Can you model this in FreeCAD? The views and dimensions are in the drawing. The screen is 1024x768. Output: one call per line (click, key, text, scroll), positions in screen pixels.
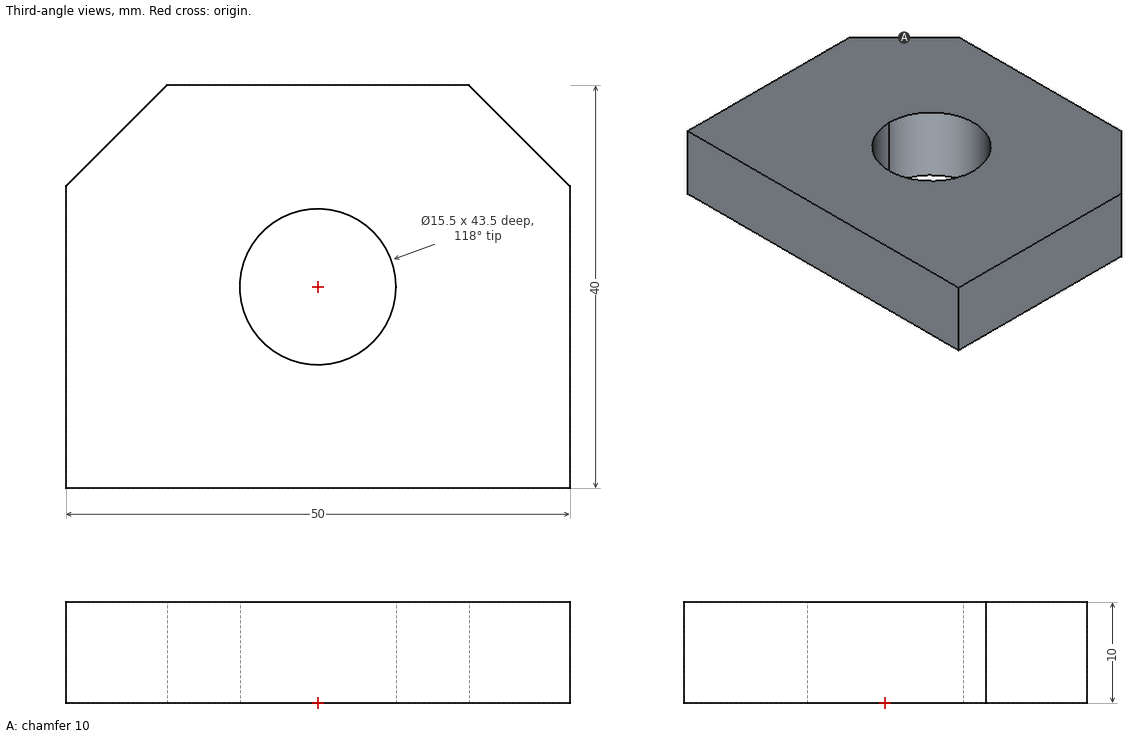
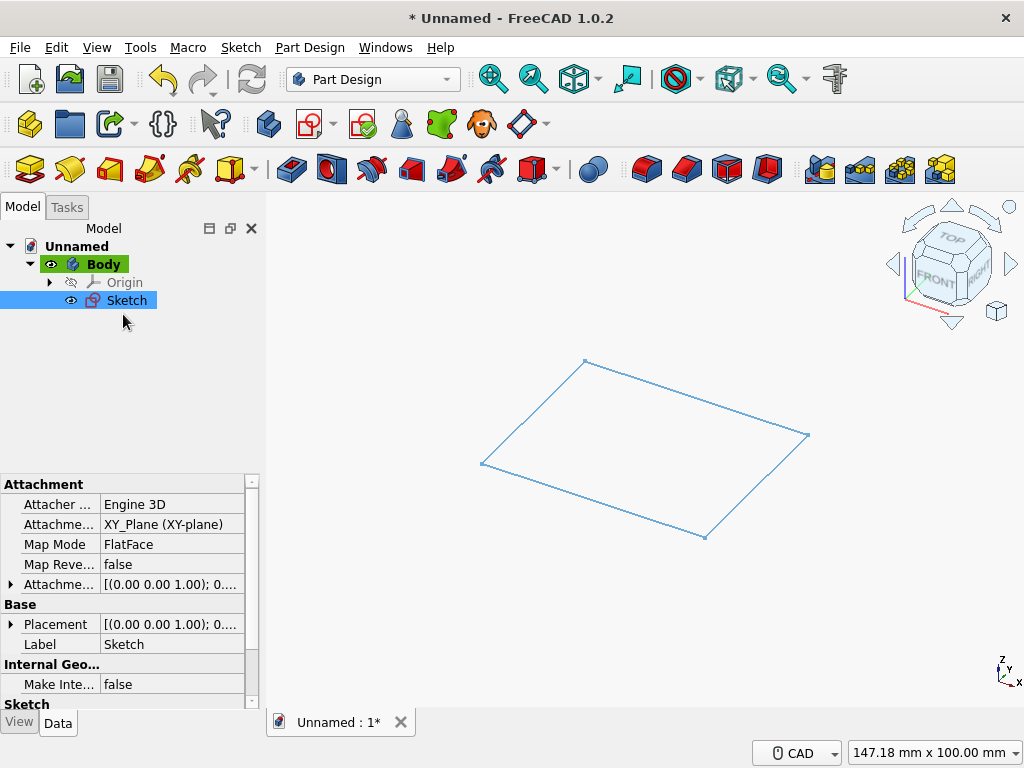
click(30, 170)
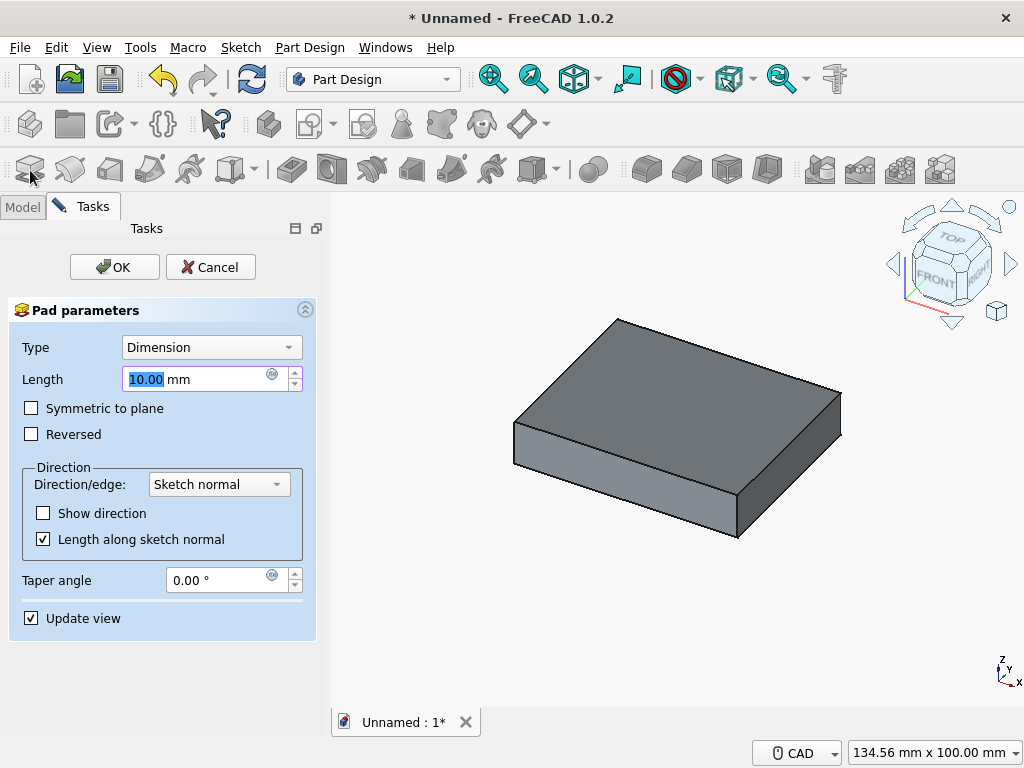
text(10)
key(Tab)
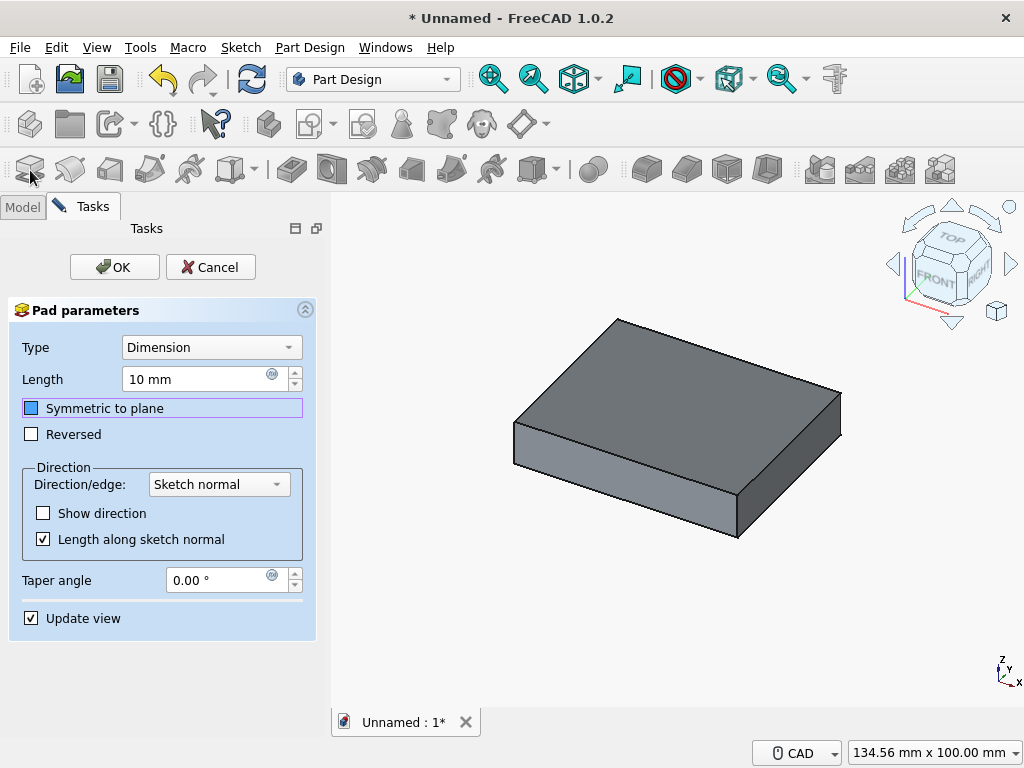
click(115, 267)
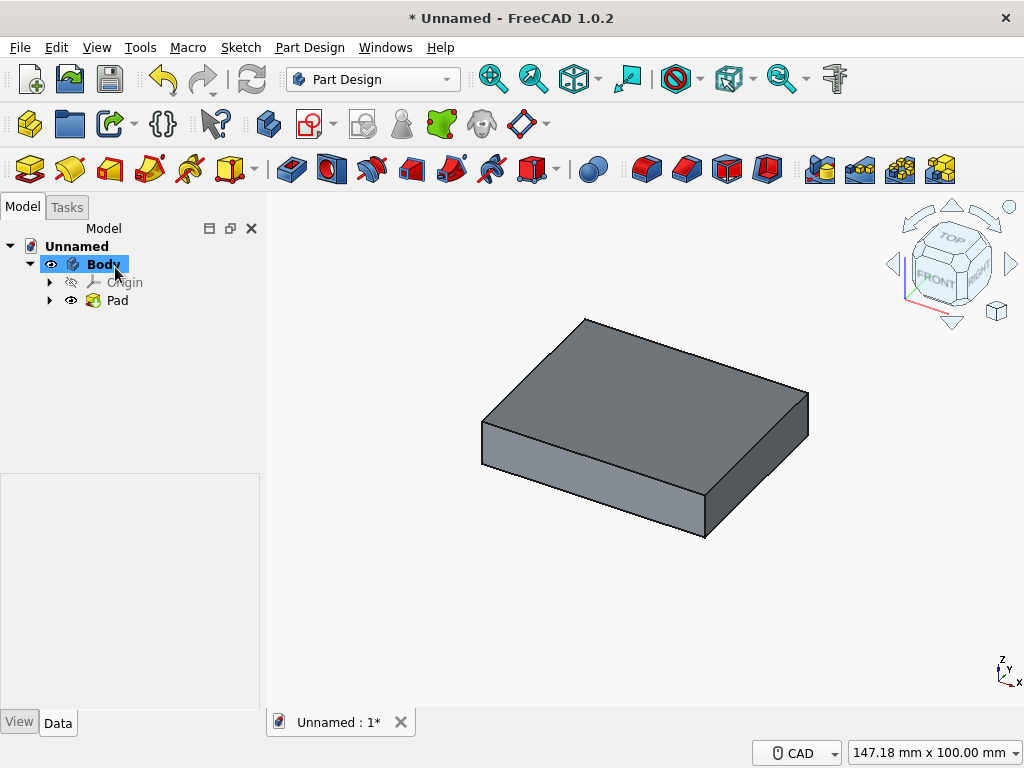
key(v)
key(f)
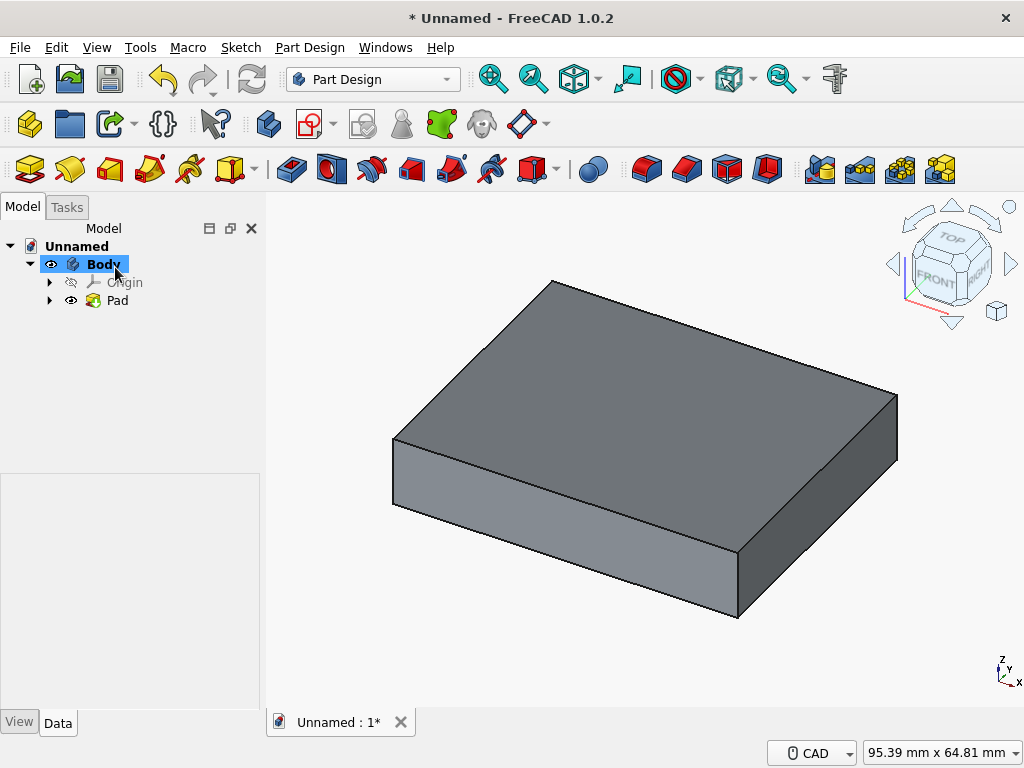
key(0)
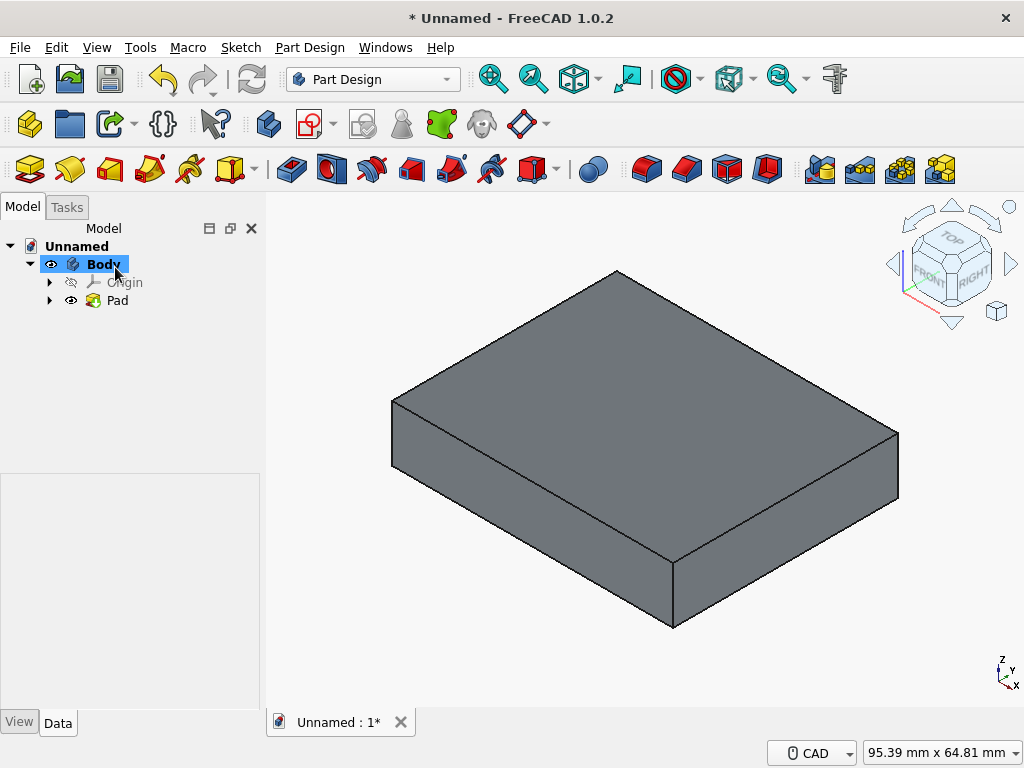
key(2)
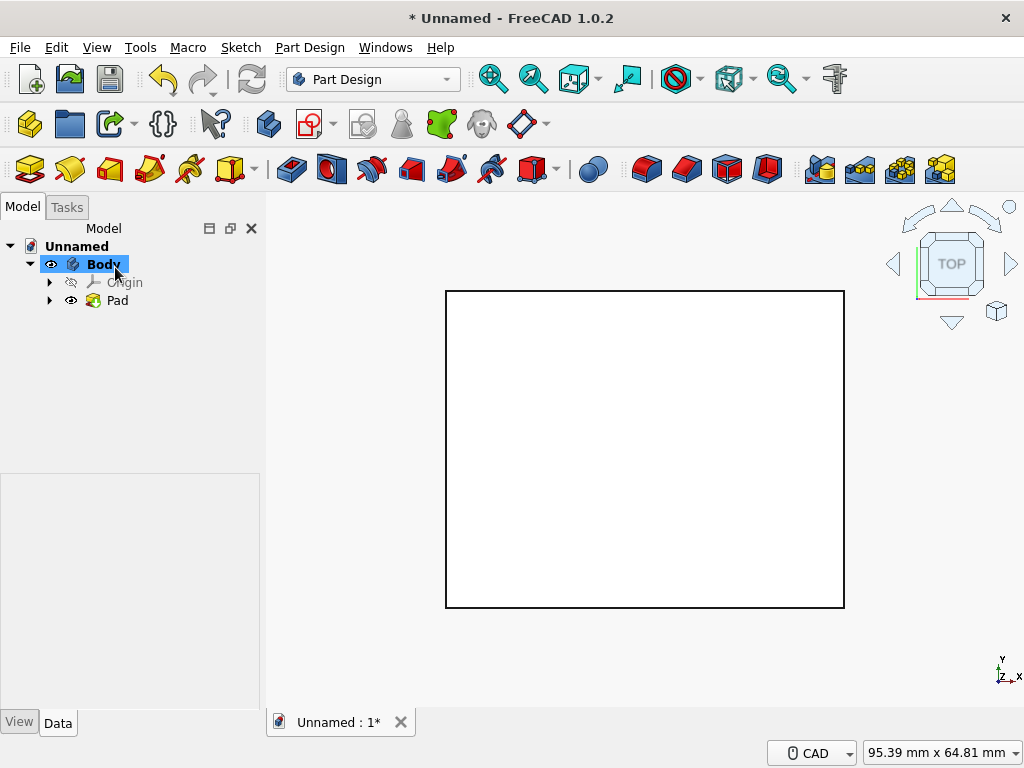
key(1)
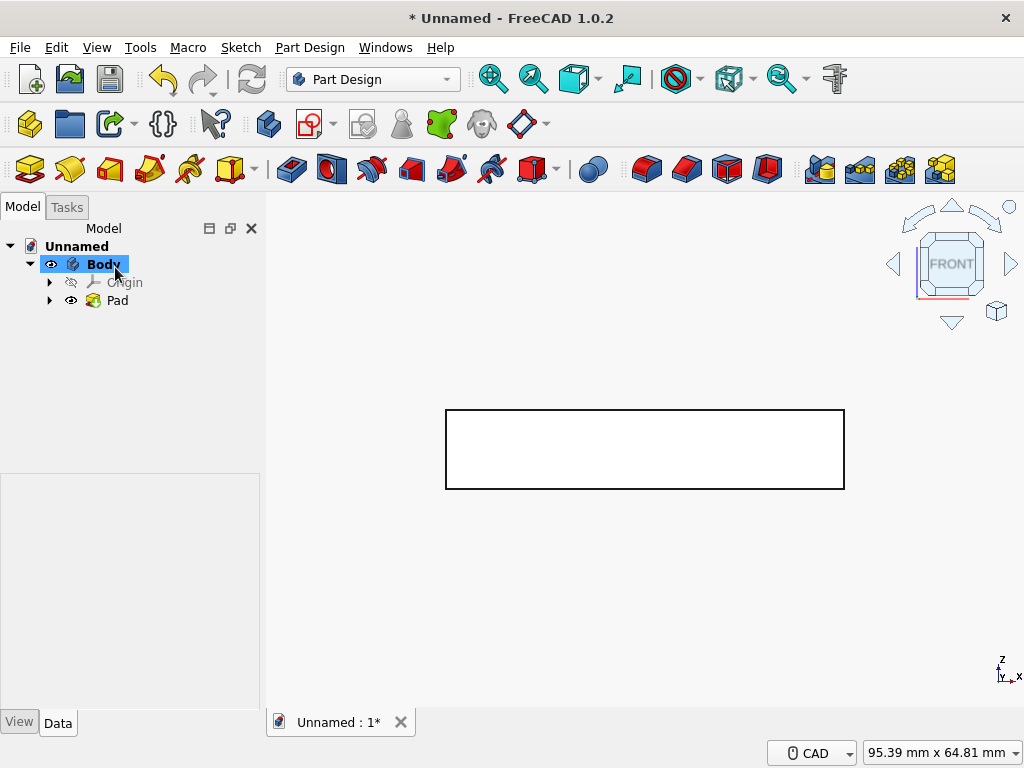
key(3)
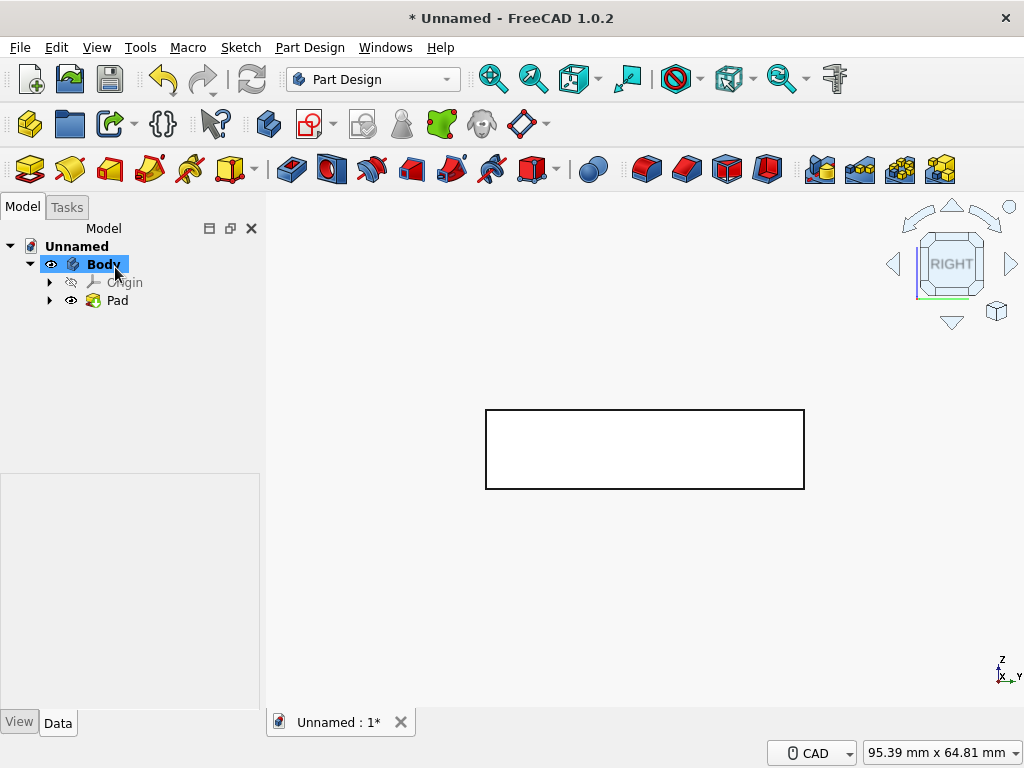
key(v)
key(f)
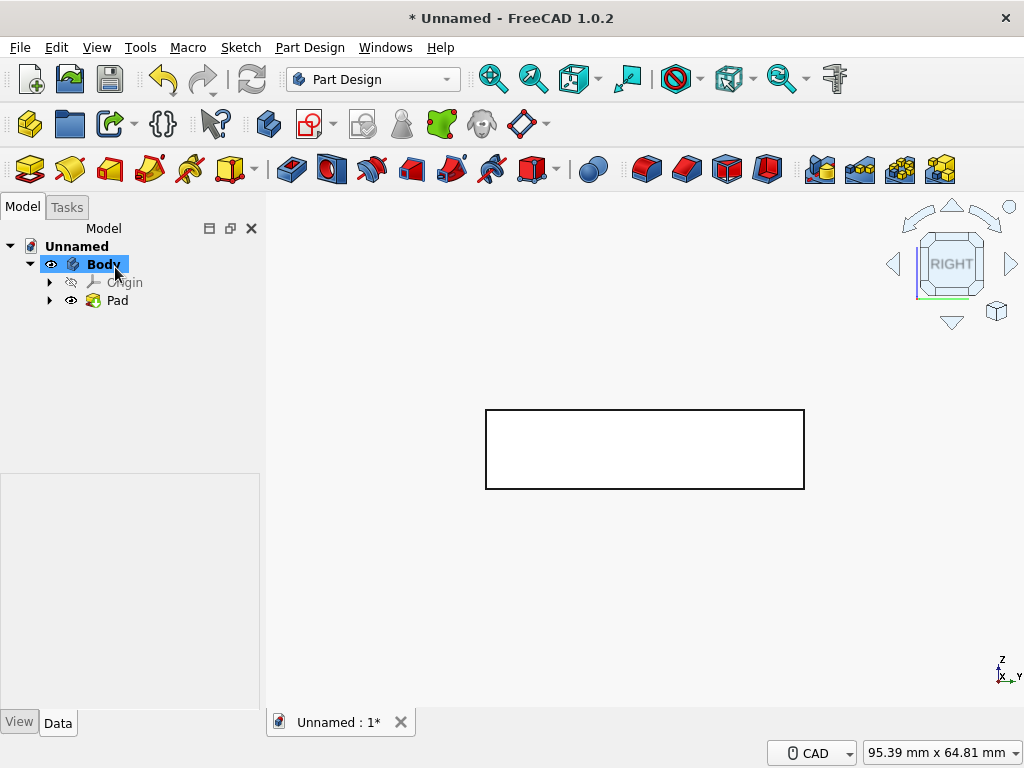
click(804, 448)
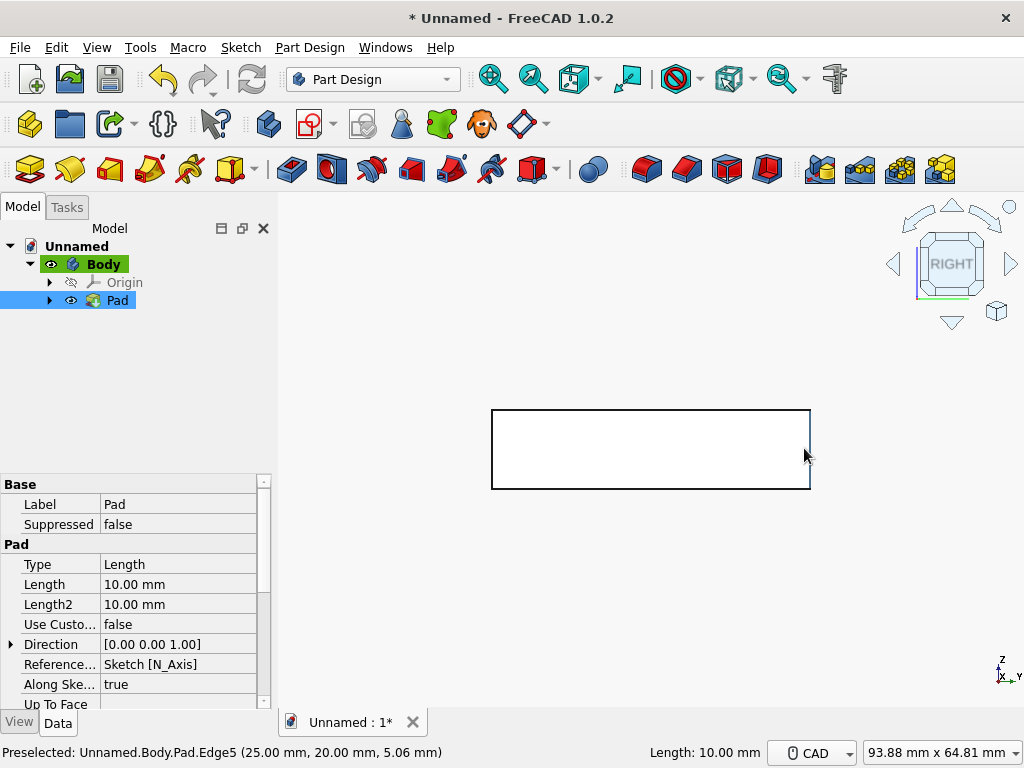
key(5)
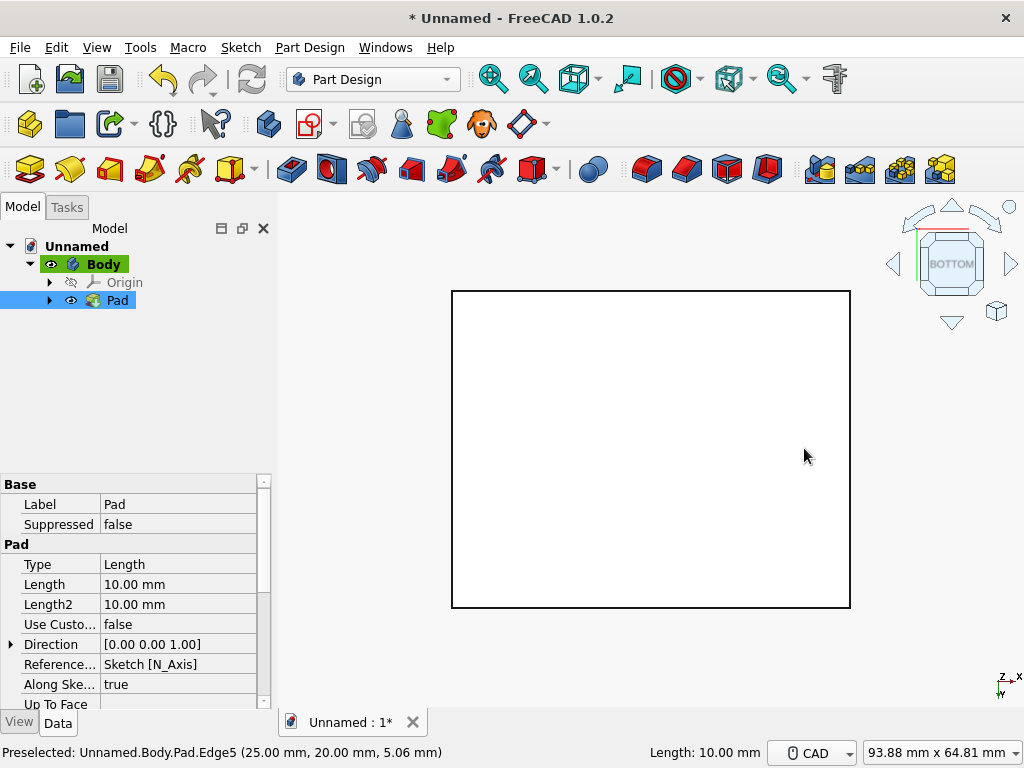
key(4)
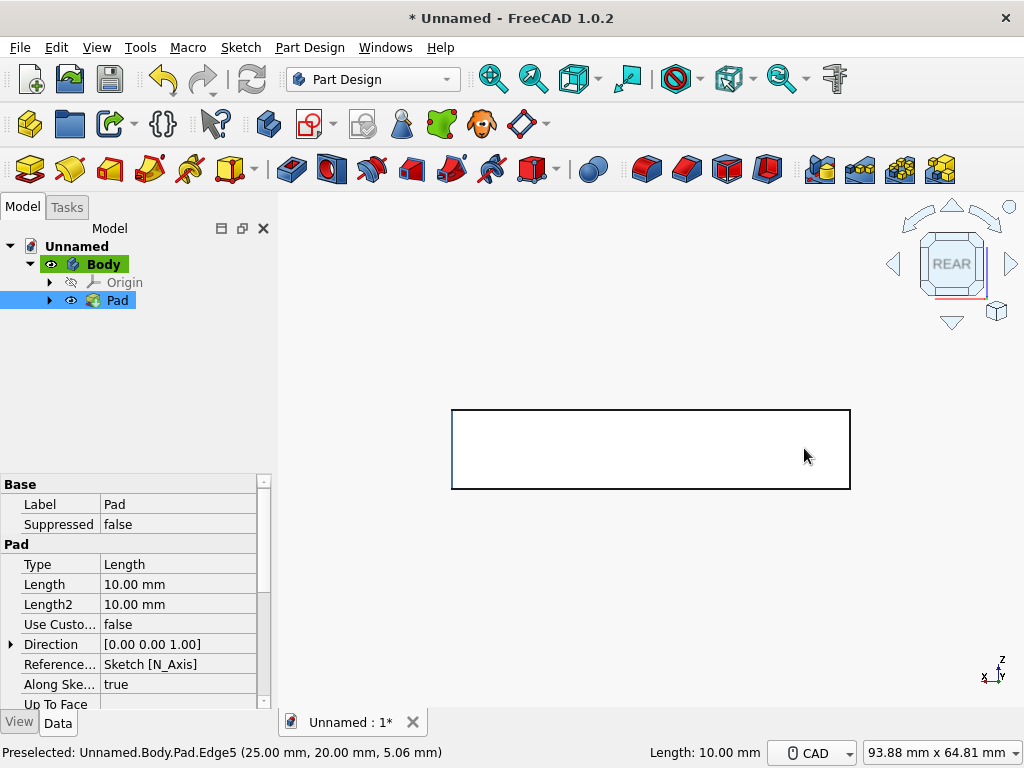
click(850, 449, ctrl)